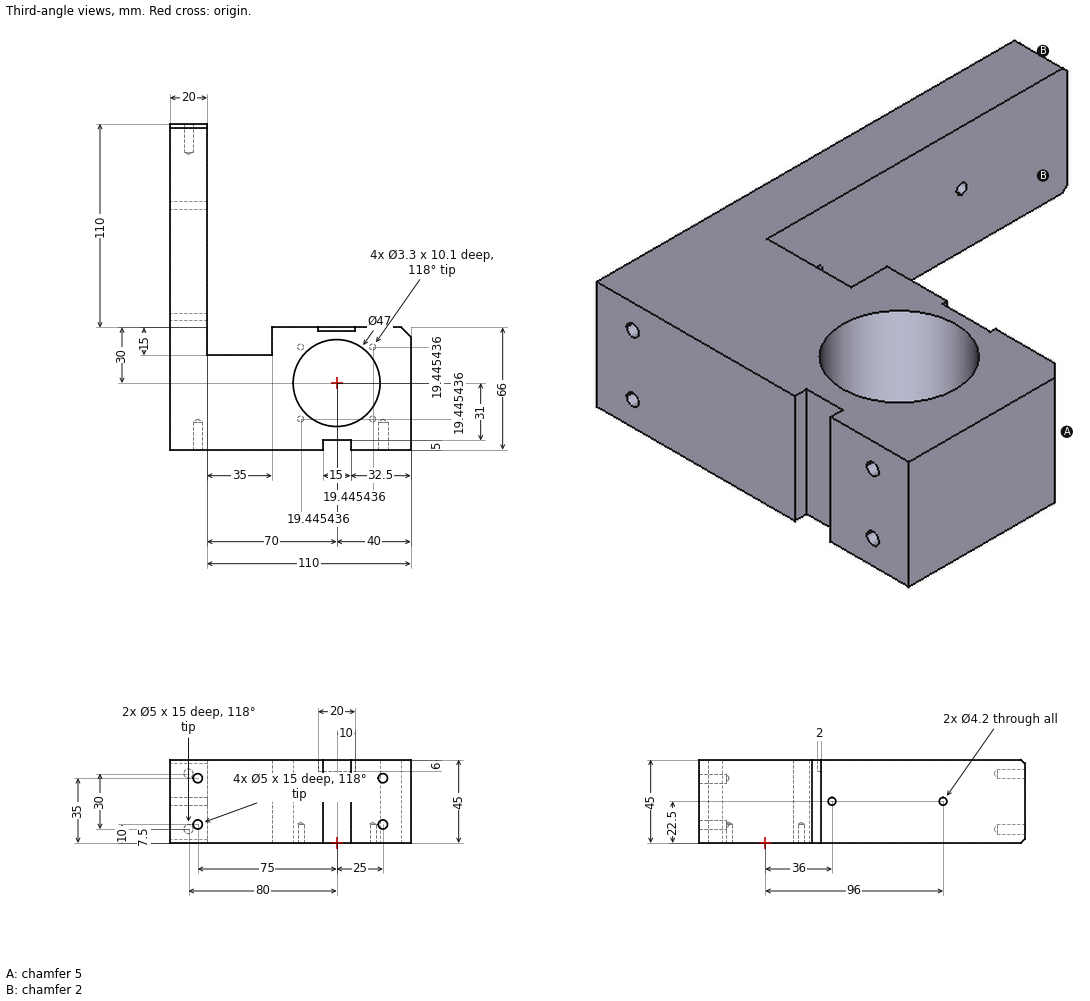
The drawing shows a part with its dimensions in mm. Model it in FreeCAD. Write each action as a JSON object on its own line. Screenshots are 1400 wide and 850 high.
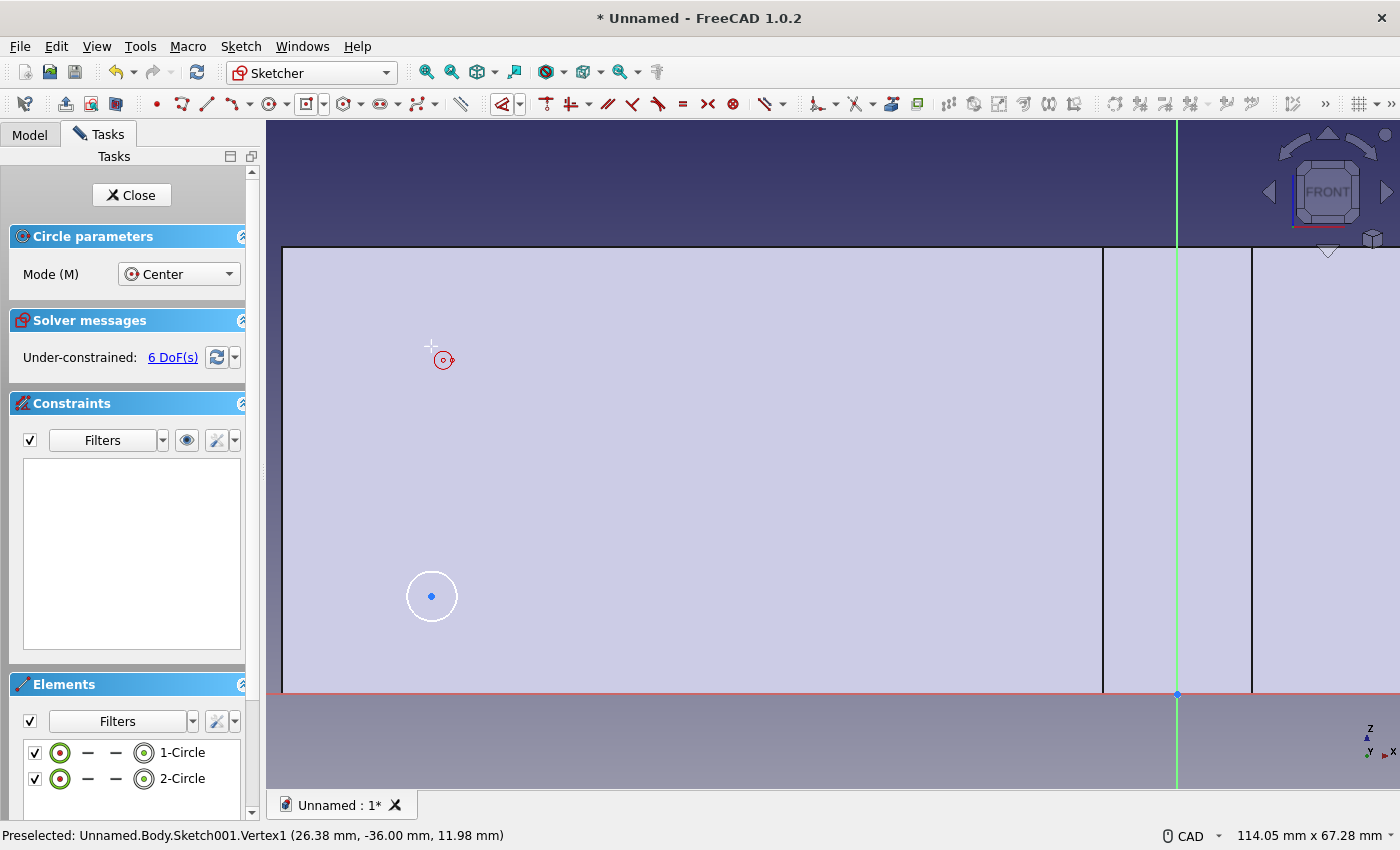
{"action": "left_click", "coordinate": [432, 346]}
{"action": "left_click", "coordinate": [449, 329]}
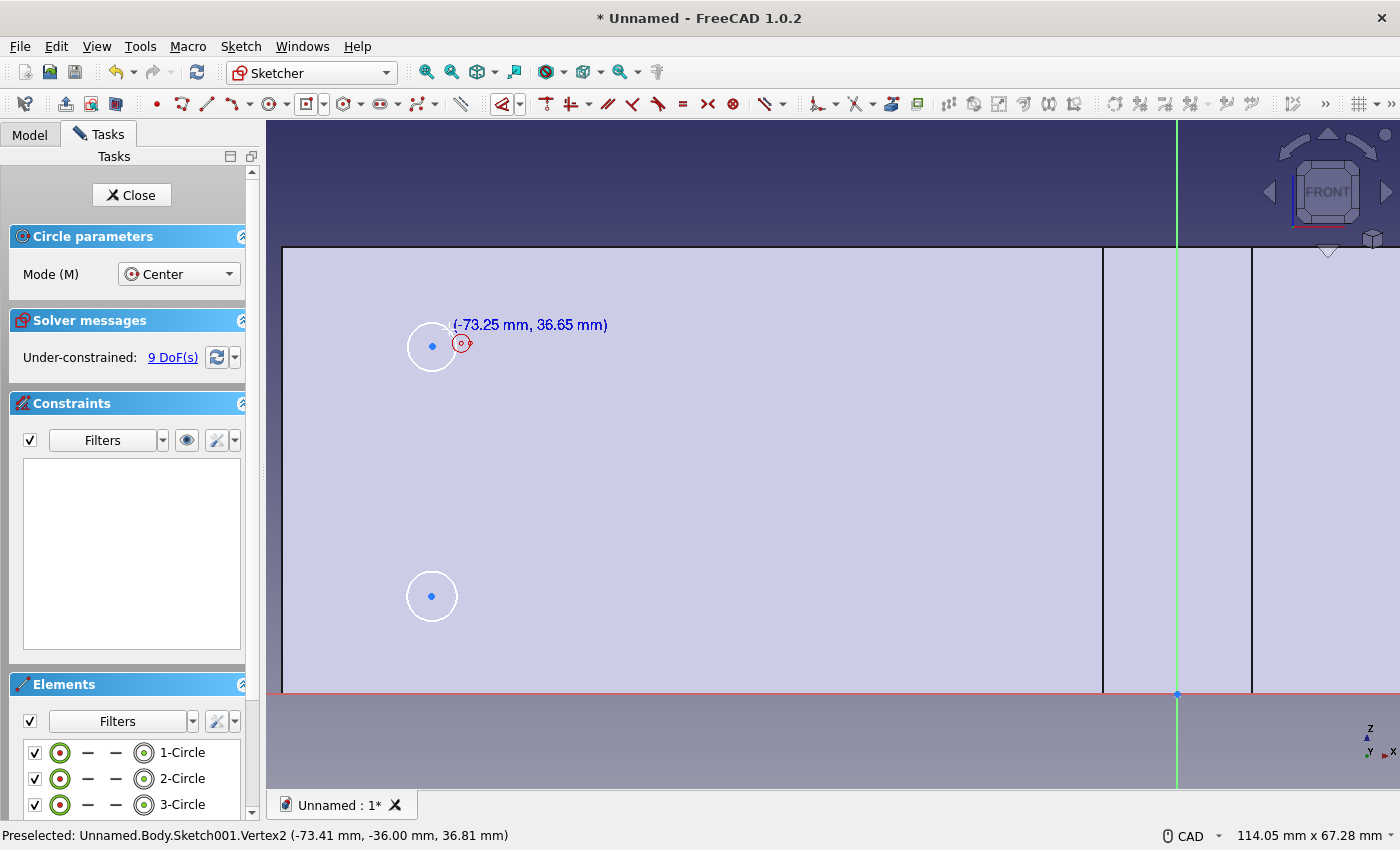
{"action": "scroll", "coordinate": [431, 346], "scroll_direction": "down", "scroll_amount": 2}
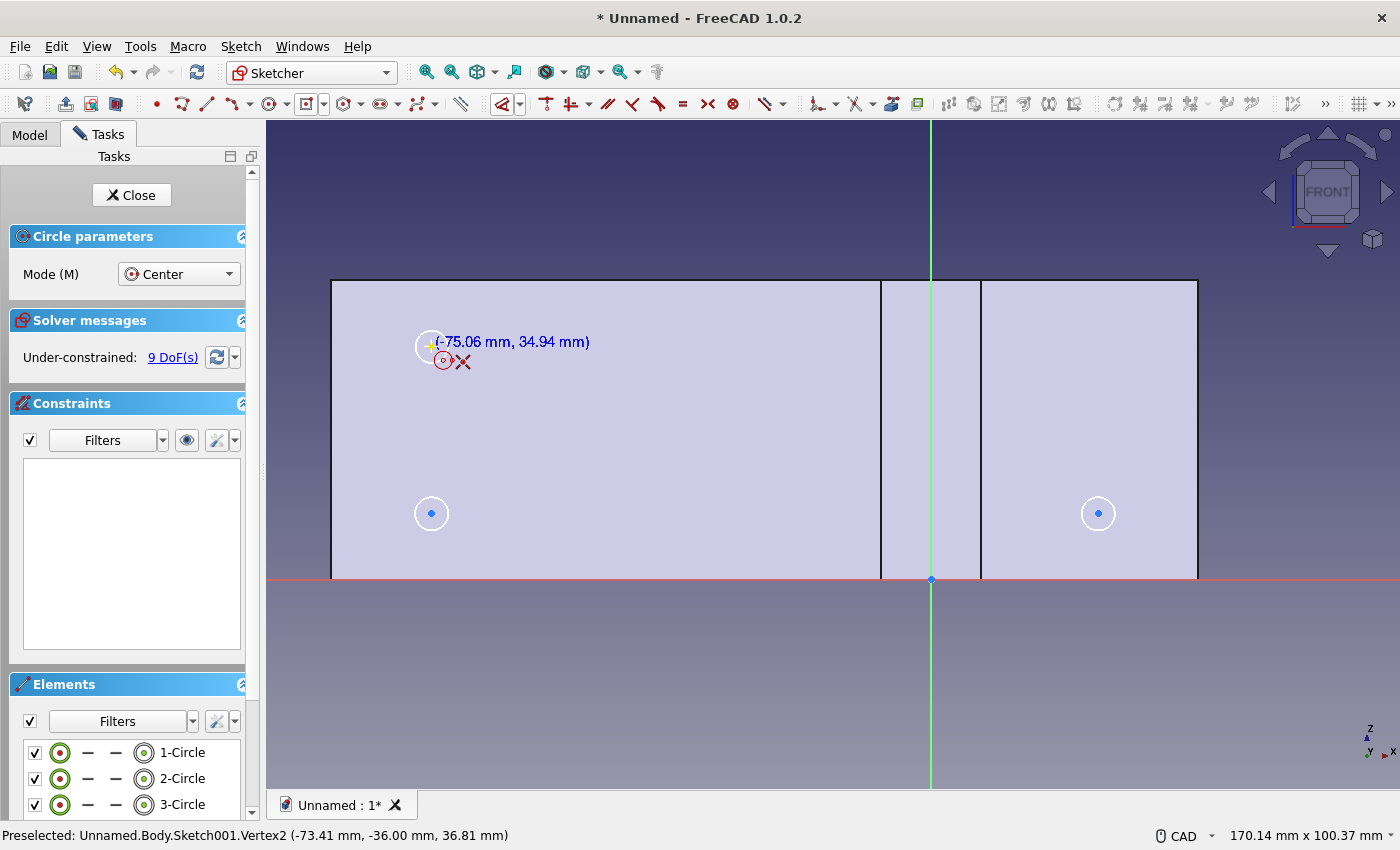
{"action": "scroll", "coordinate": [1098, 346], "scroll_direction": "up", "scroll_amount": 2}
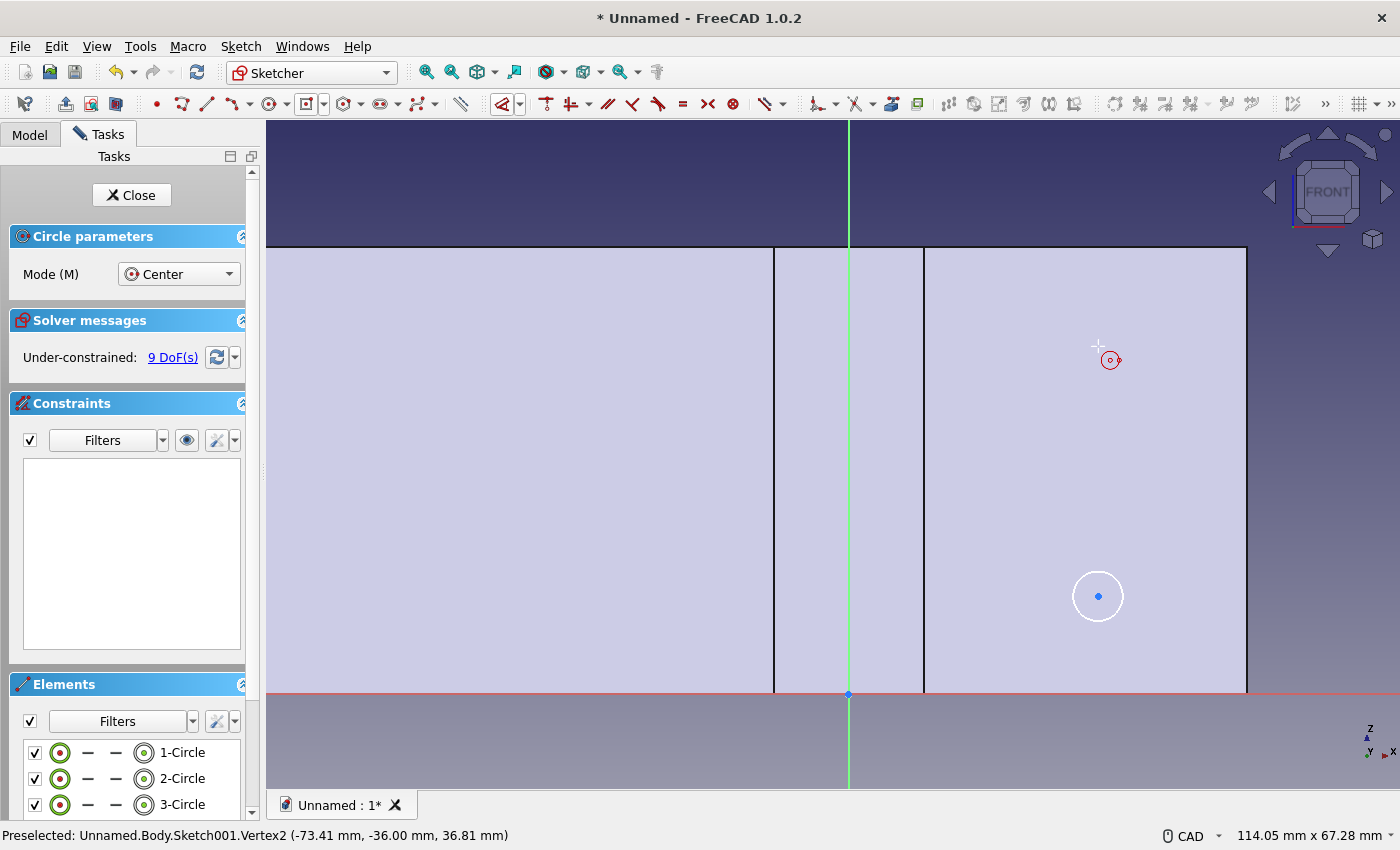
{"action": "left_click", "coordinate": [1098, 346]}
{"action": "left_click", "coordinate": [1115, 329]}
{"action": "key", "text": "Escape"}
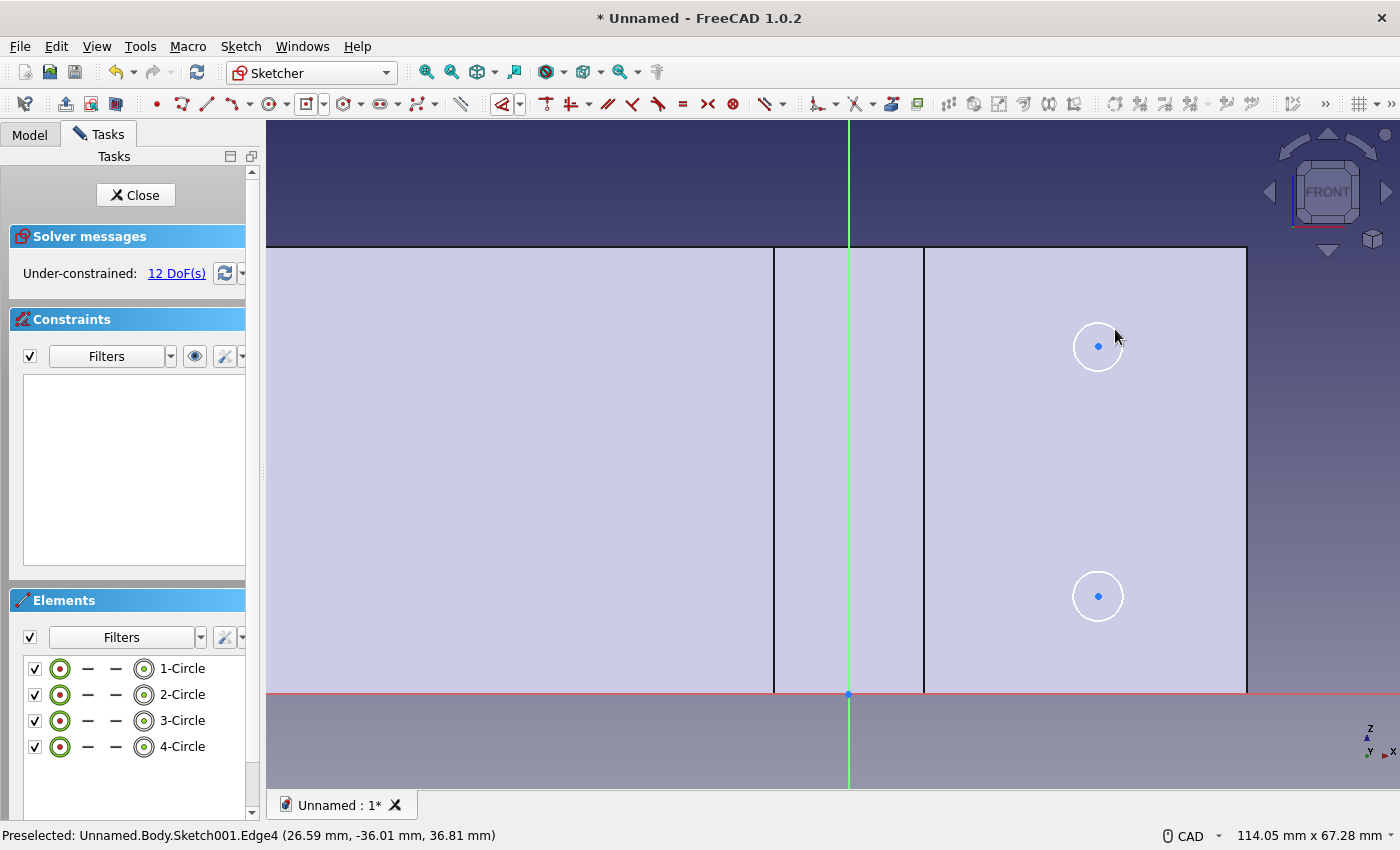
{"action": "scroll", "coordinate": [1098, 346], "scroll_direction": "down", "scroll_amount": 2}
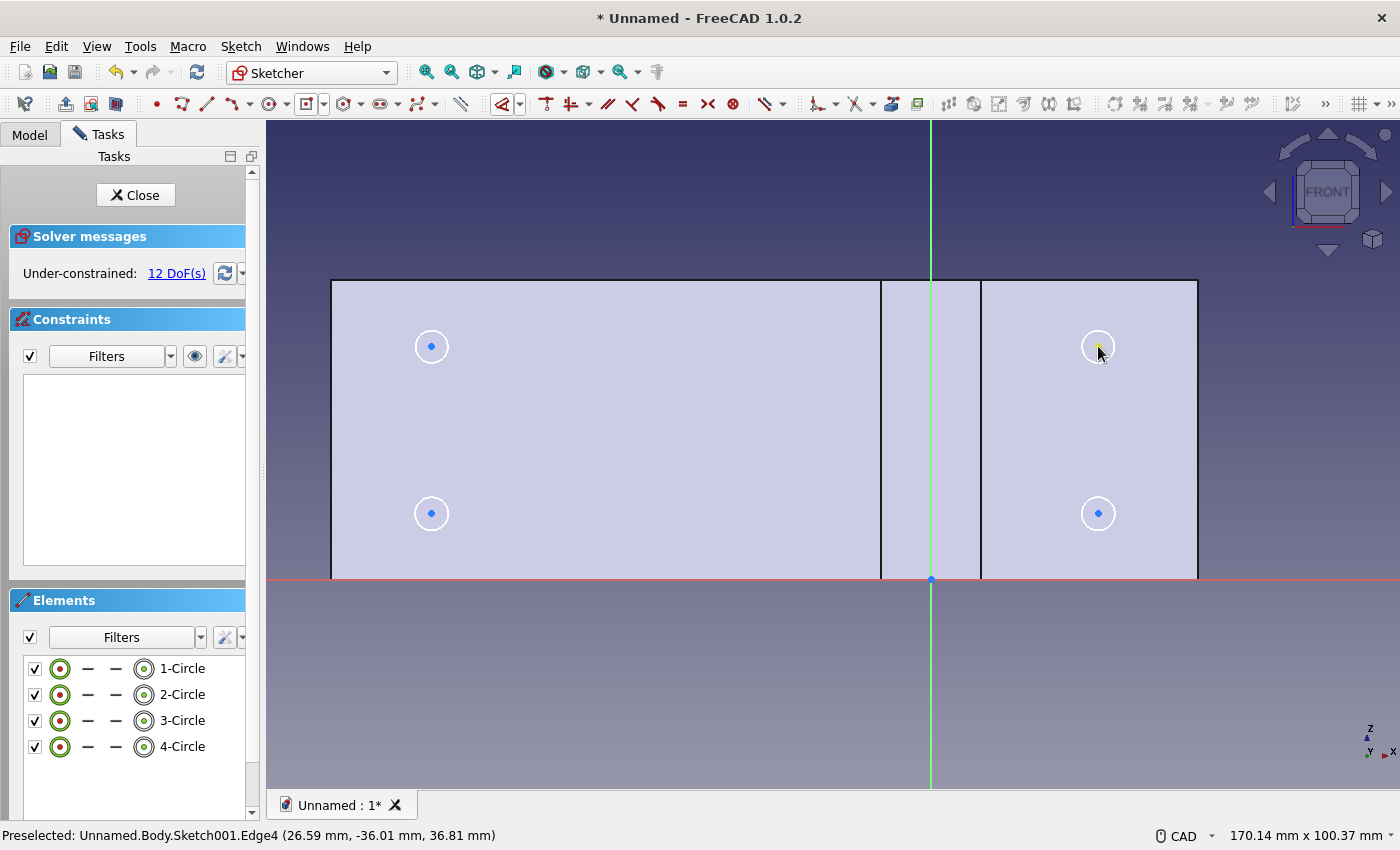
{"action": "left_click", "coordinate": [443, 502]}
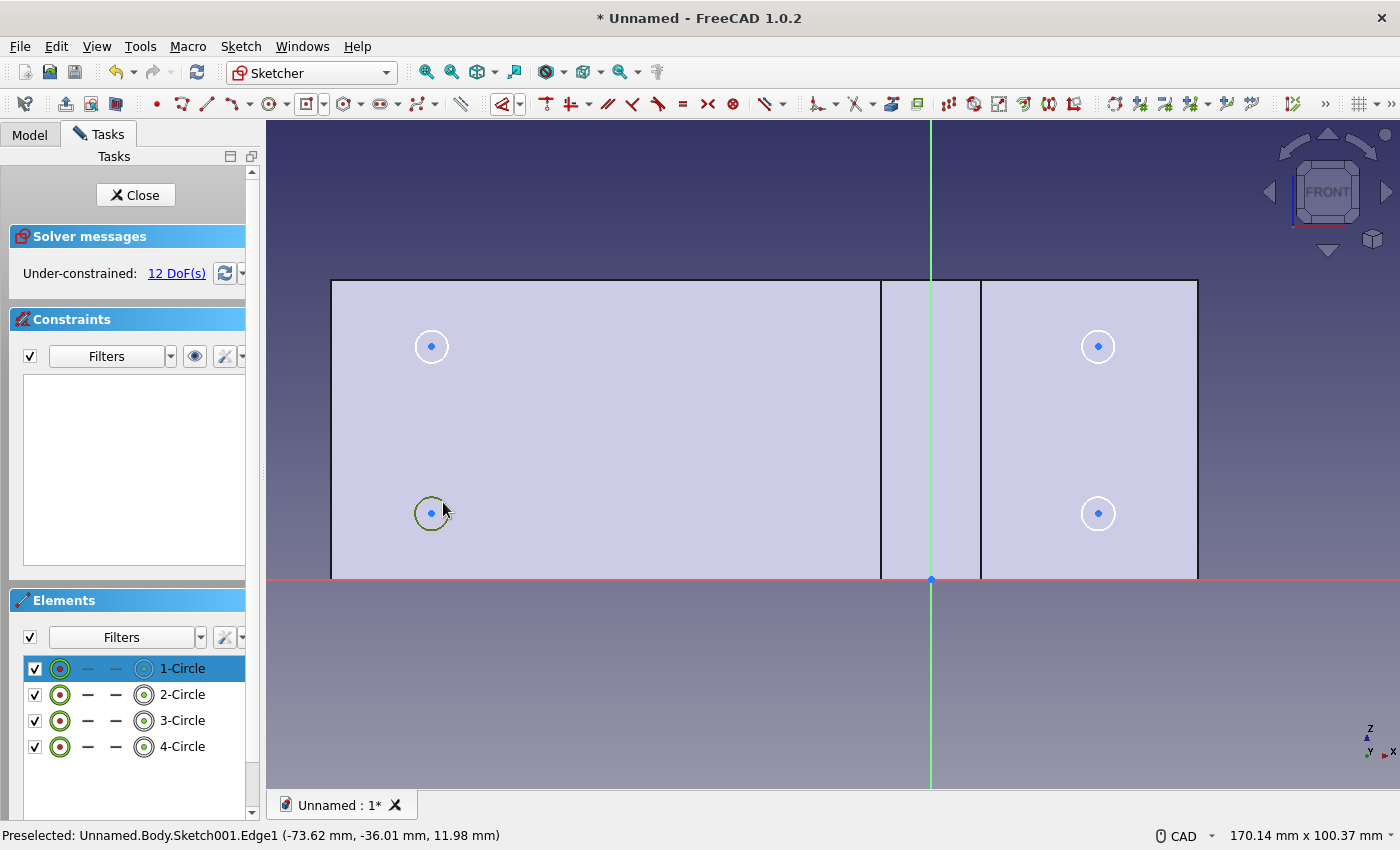
{"action": "left_click", "coordinate": [1110, 502]}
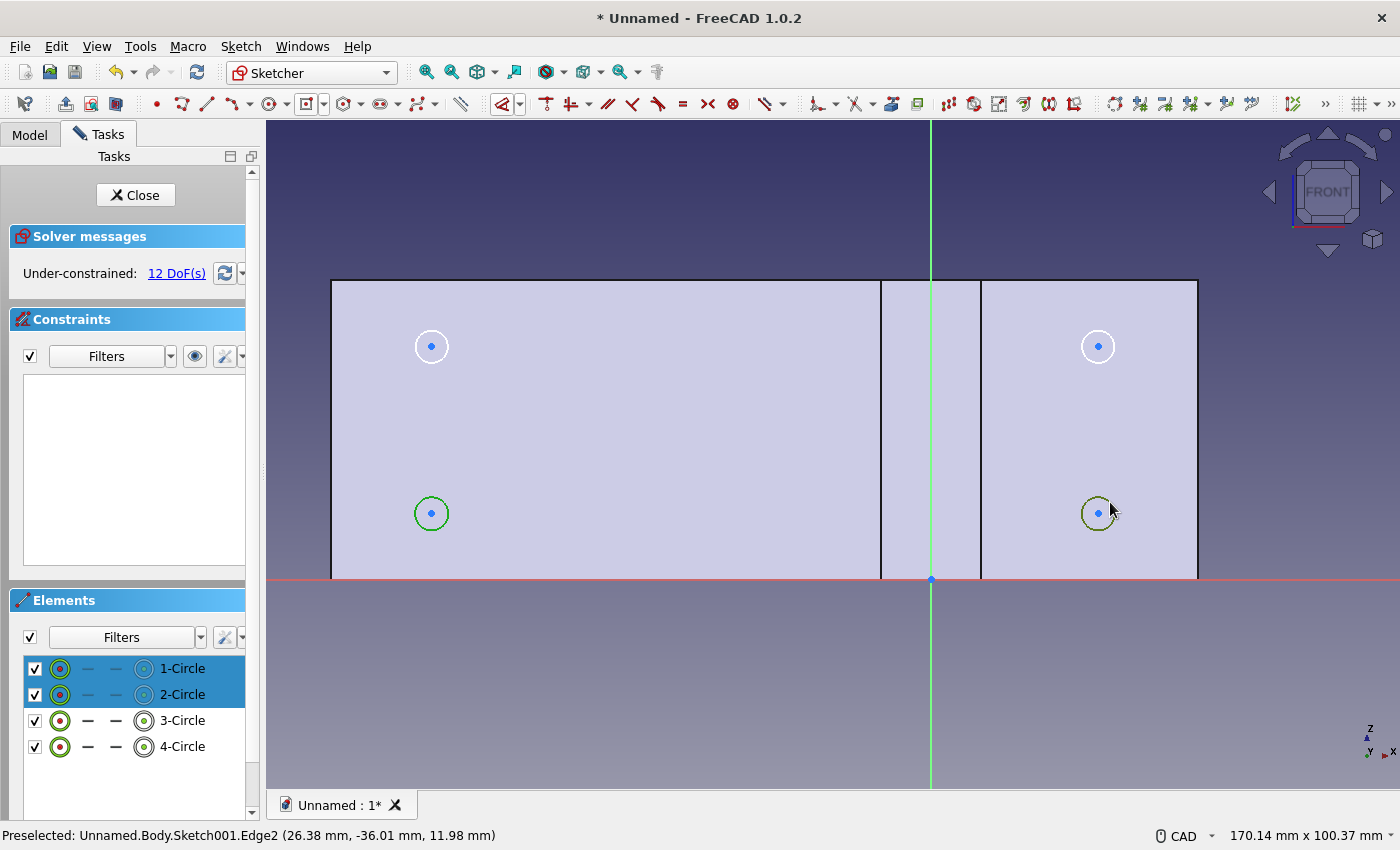
{"action": "left_click", "coordinate": [443, 335]}